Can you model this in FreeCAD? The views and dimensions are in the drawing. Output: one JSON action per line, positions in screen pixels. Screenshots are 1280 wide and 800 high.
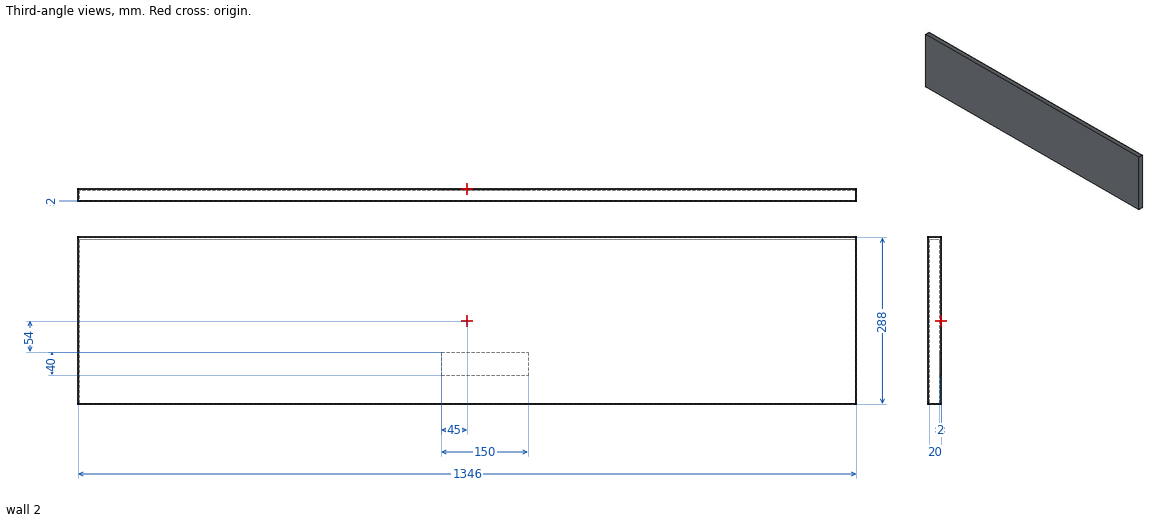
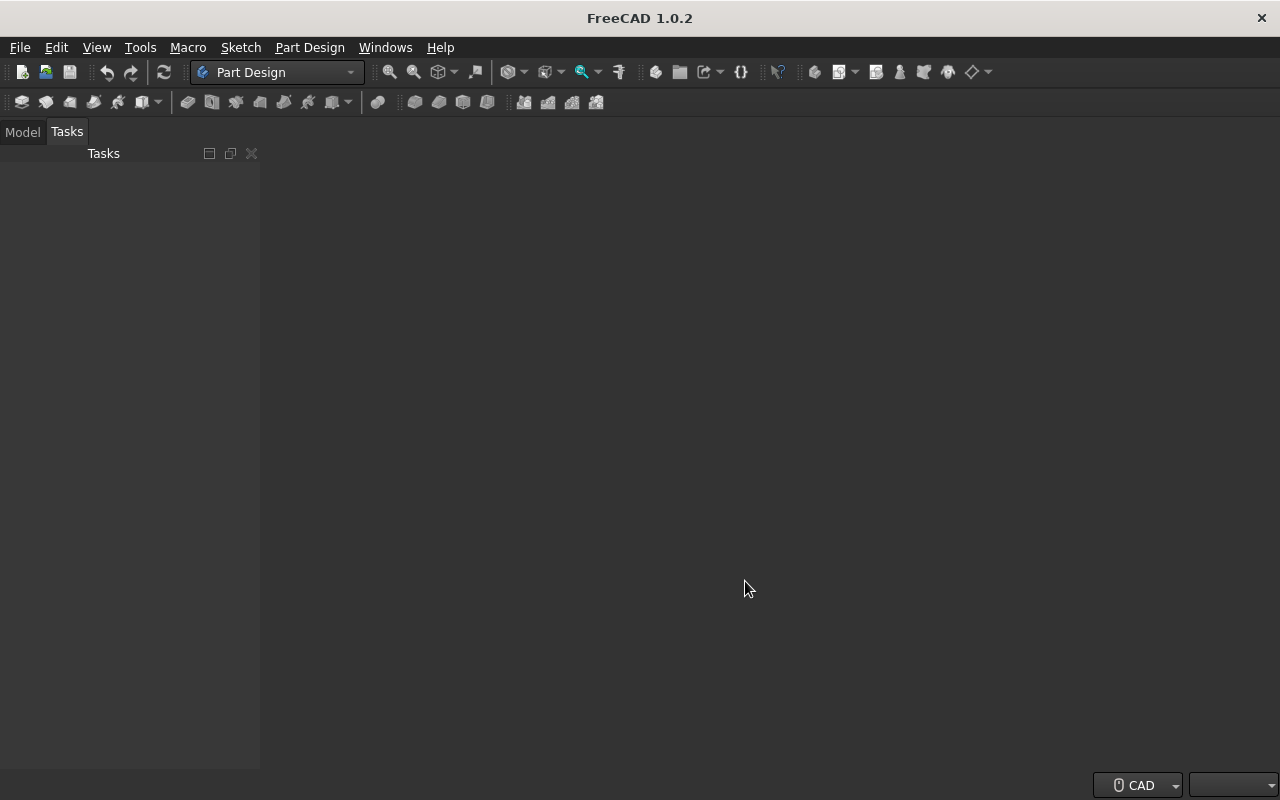
{"action": "key", "text": "ctrl+n"}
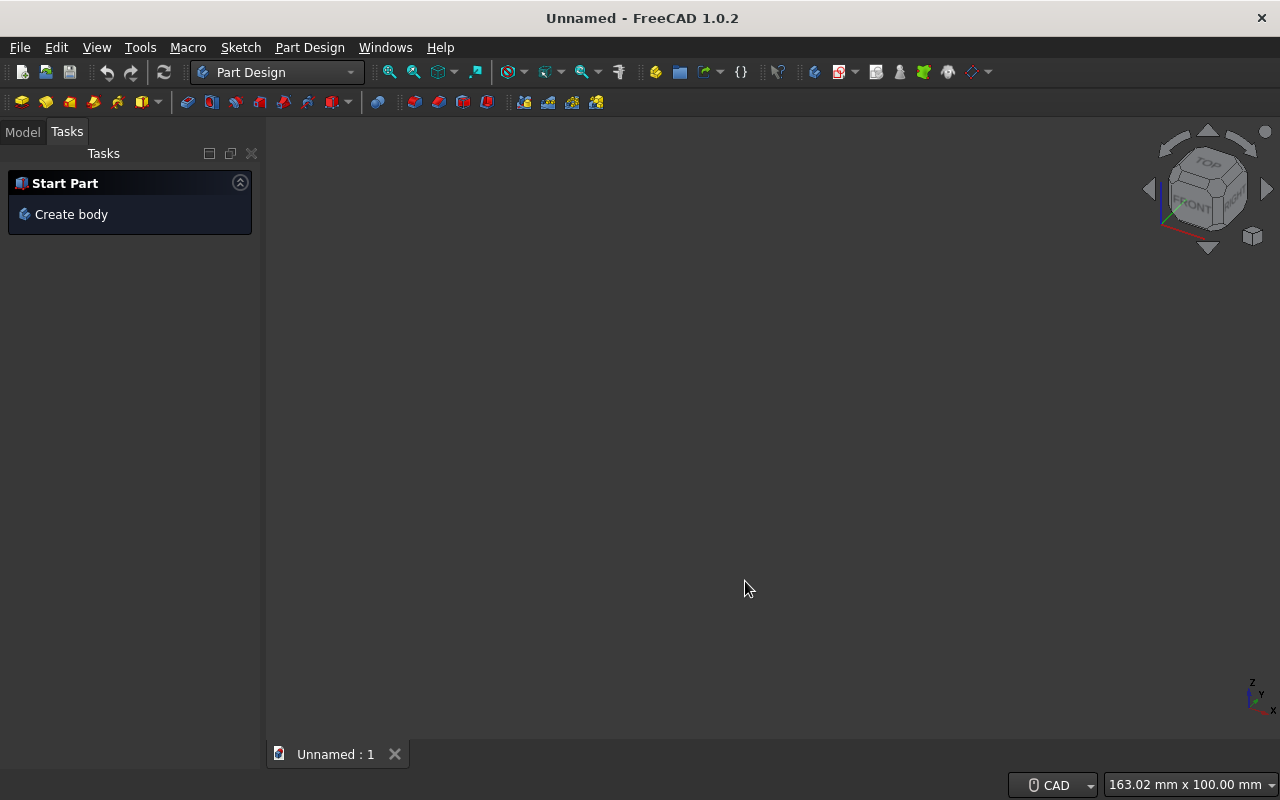
{"action": "left_click", "coordinate": [840, 72]}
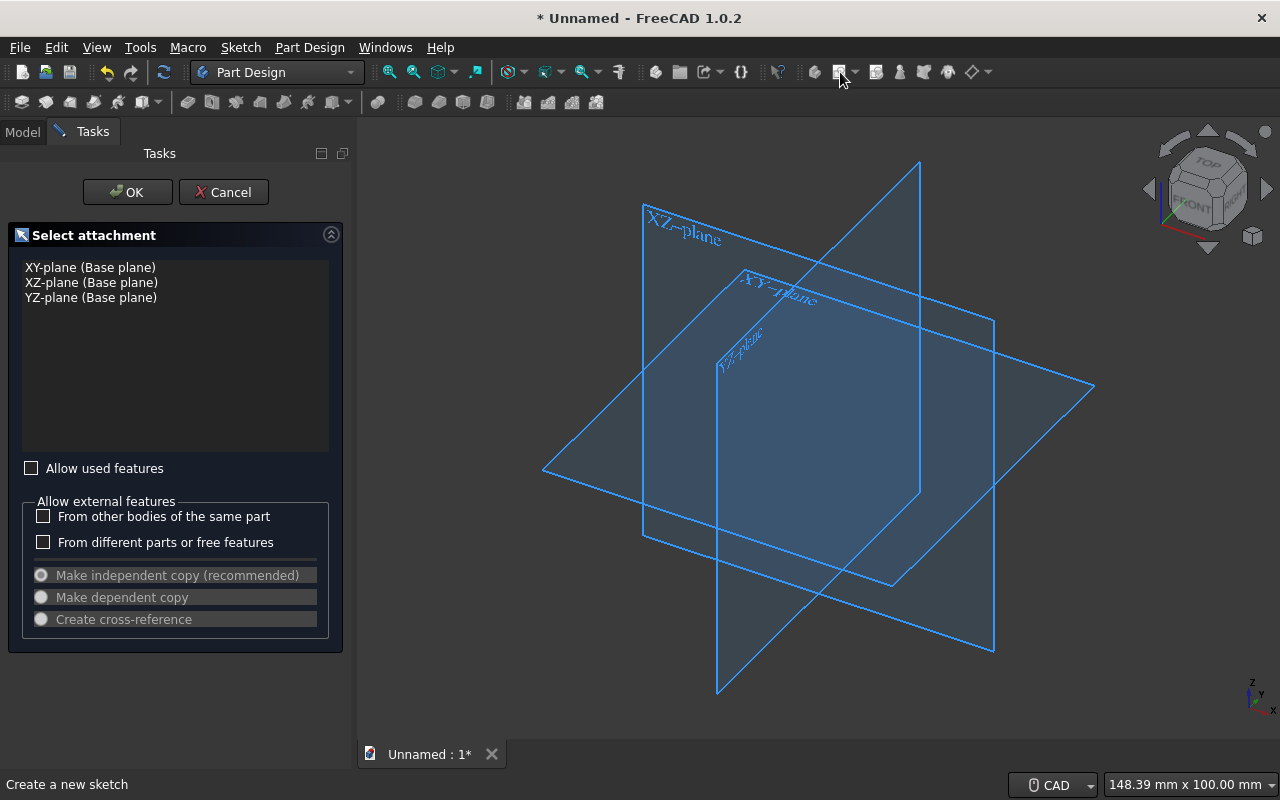
{"action": "left_click", "coordinate": [82, 282]}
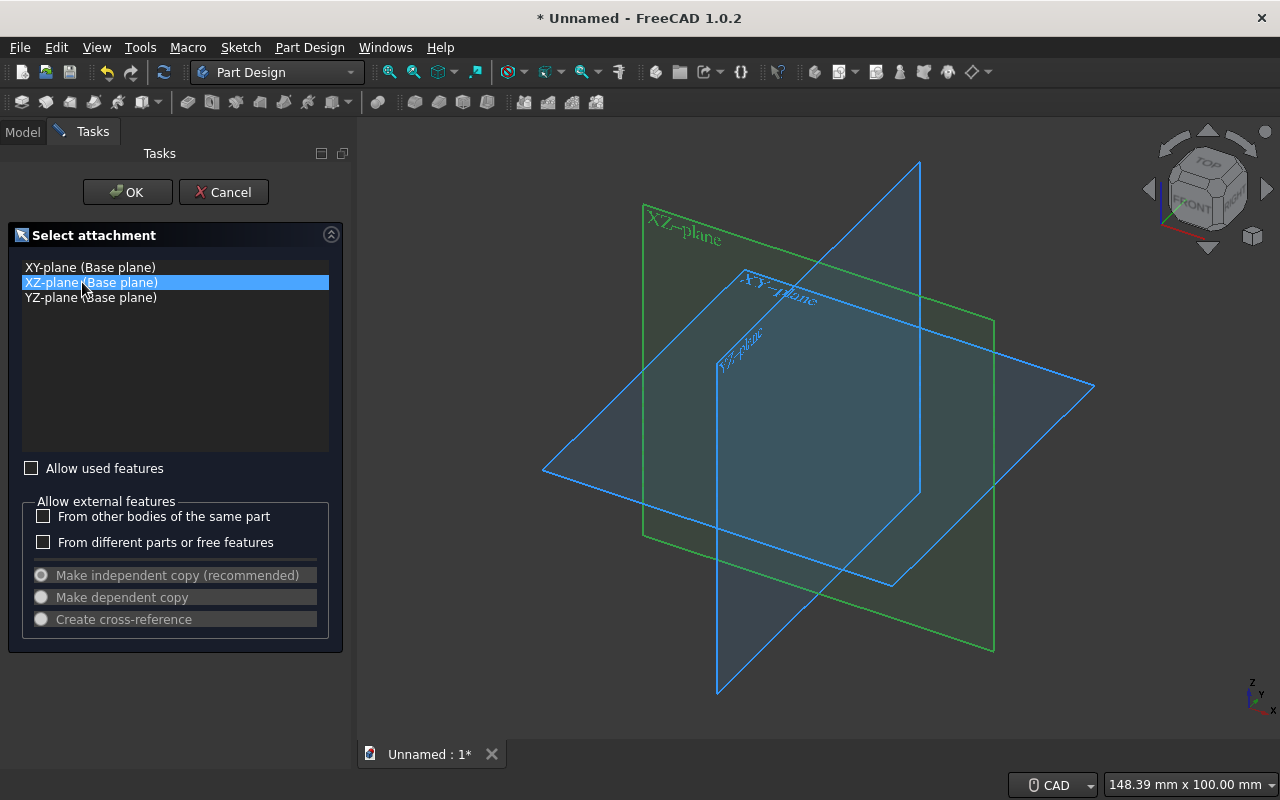
{"action": "left_click", "coordinate": [128, 192]}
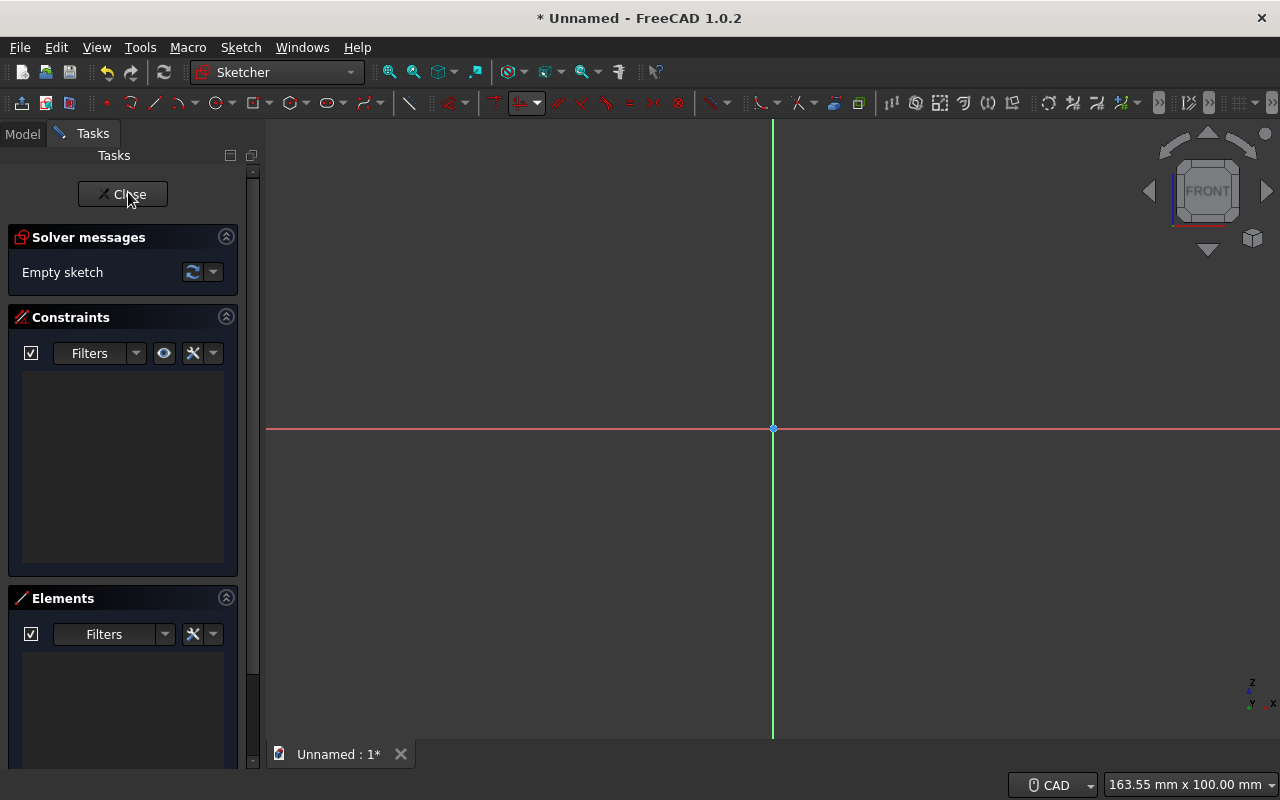
{"action": "scroll", "coordinate": [699, 429], "scroll_direction": "down", "scroll_amount": 13}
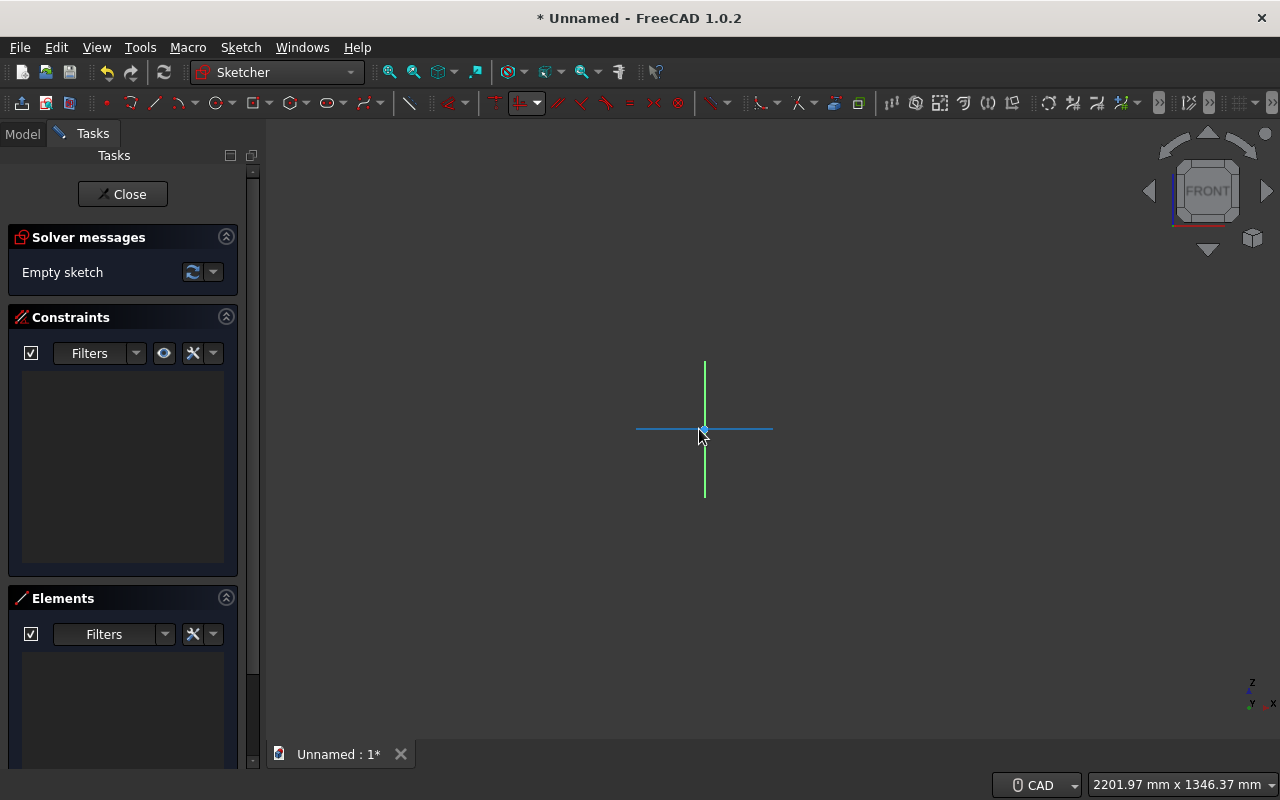
{"action": "left_click", "coordinate": [254, 104]}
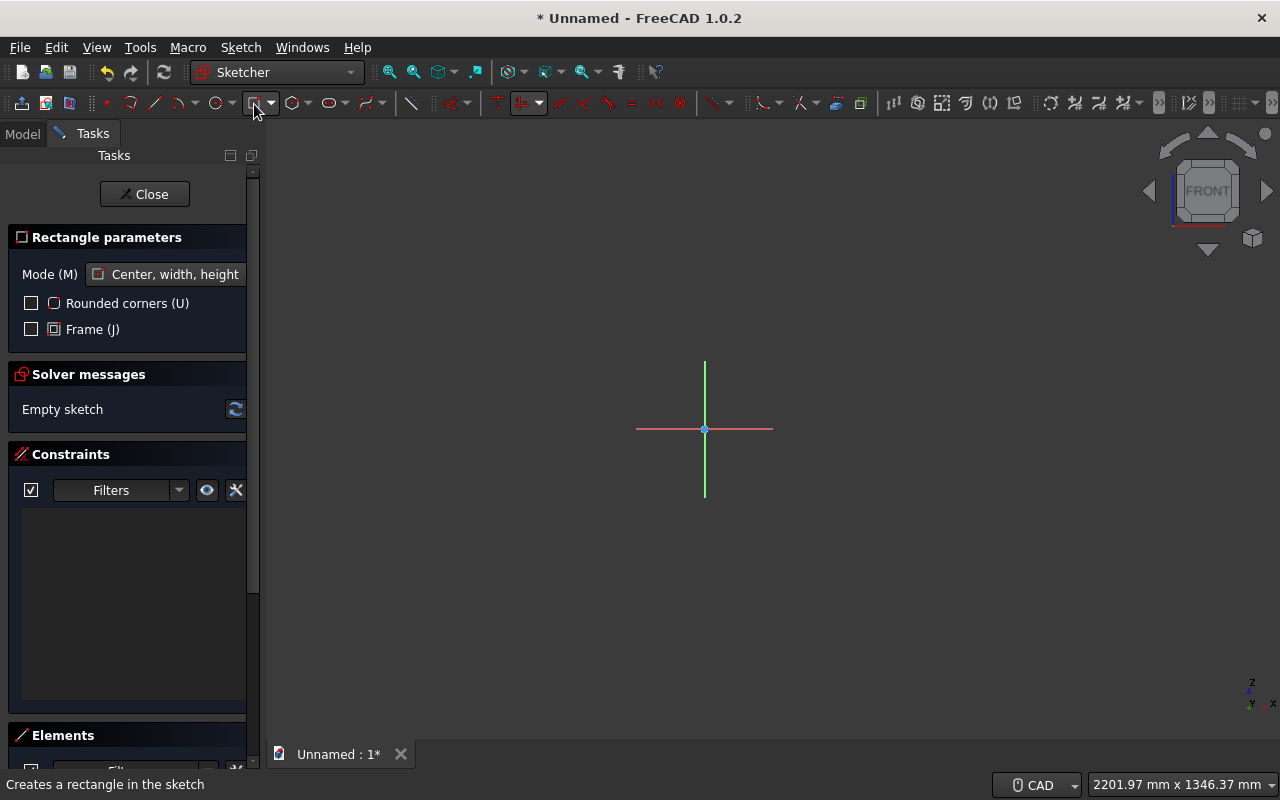
{"action": "left_click", "coordinate": [705, 429]}
{"action": "left_click", "coordinate": [1015, 363]}
{"action": "key", "text": "Escape"}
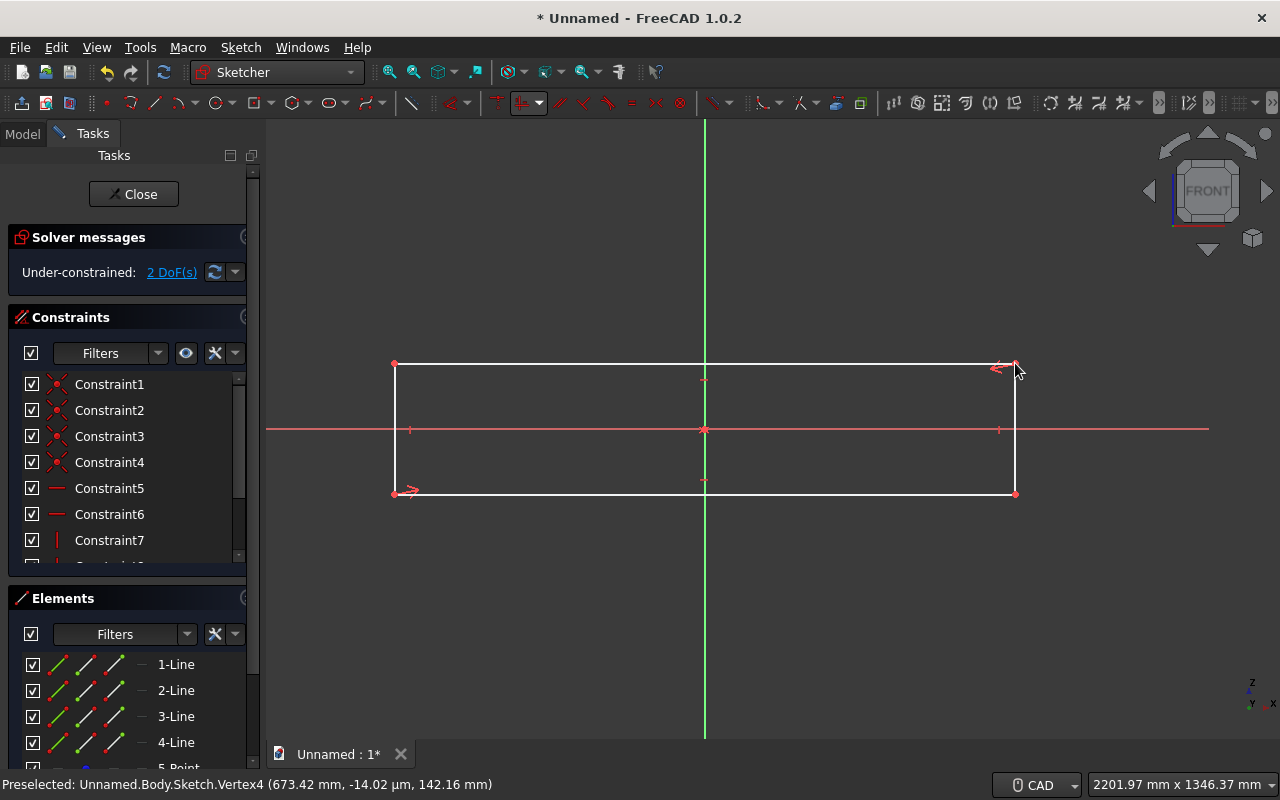
{"action": "key", "text": "d"}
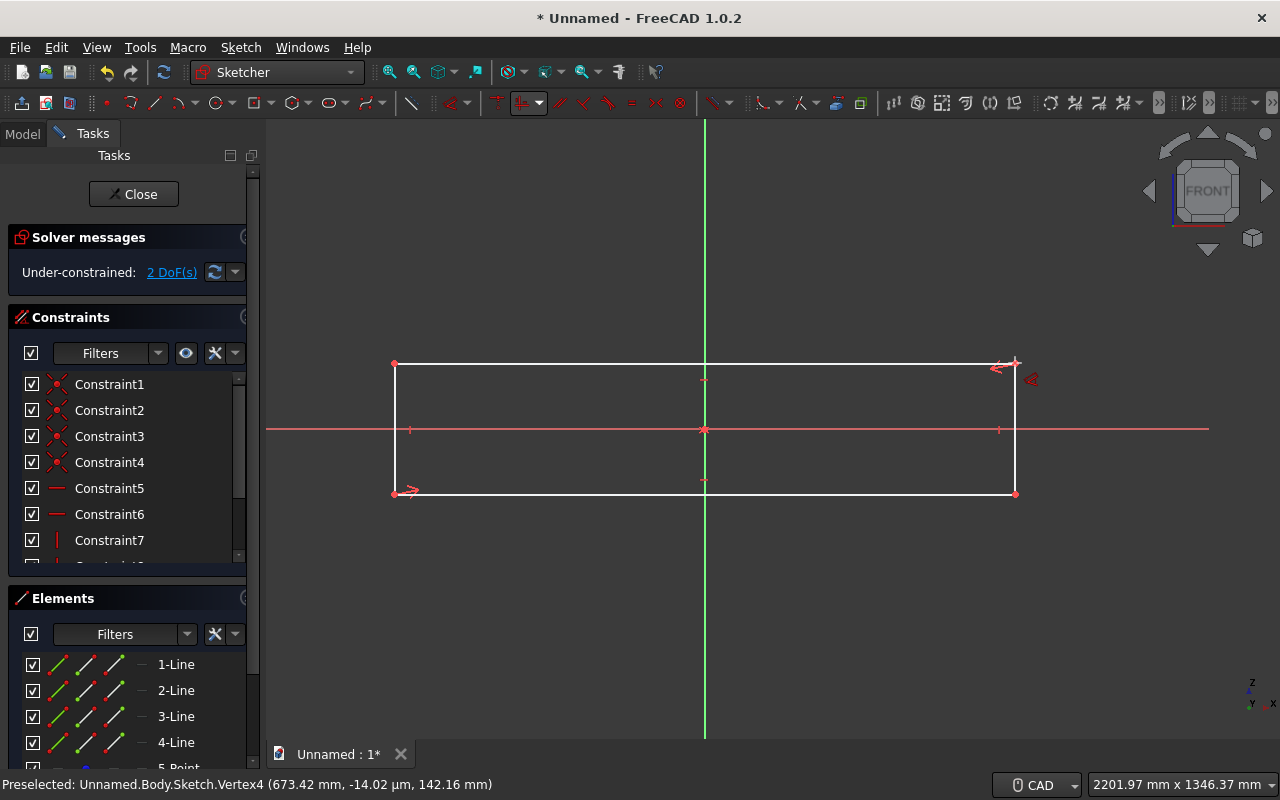
{"action": "left_click", "coordinate": [1015, 456]}
{"action": "left_click", "coordinate": [1049, 399]}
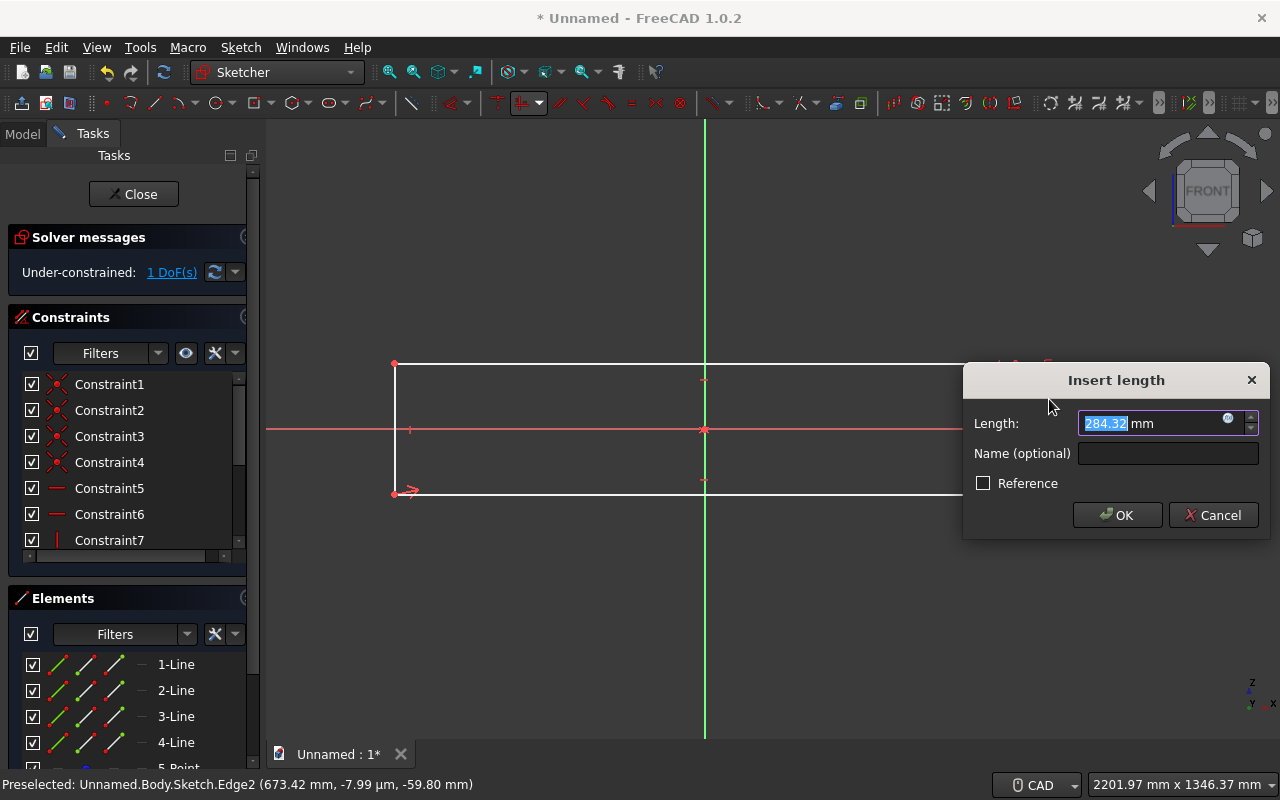
{"action": "type", "text": "288"}
{"action": "key", "text": "Return"}